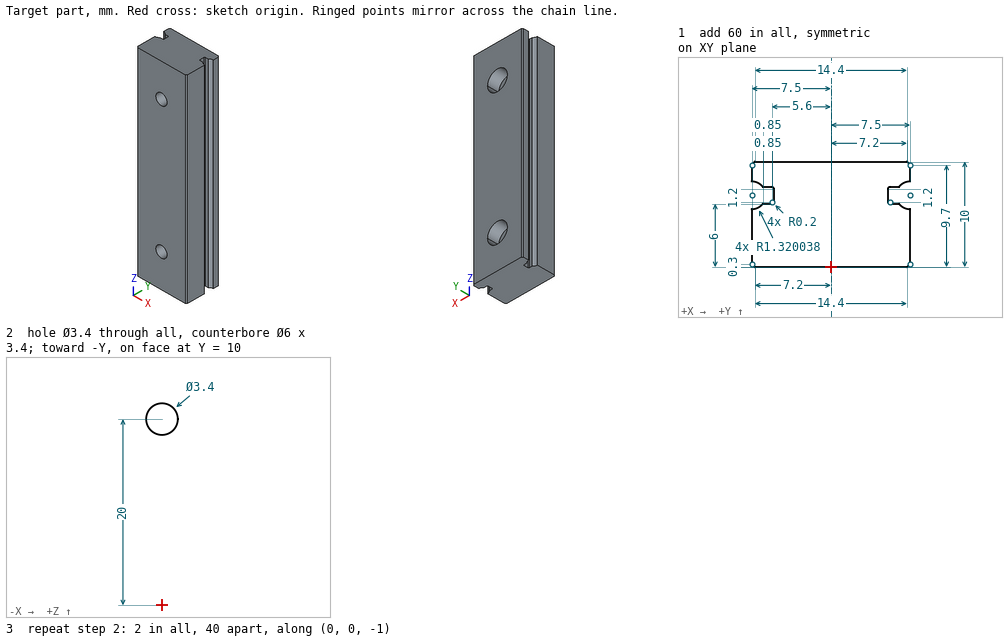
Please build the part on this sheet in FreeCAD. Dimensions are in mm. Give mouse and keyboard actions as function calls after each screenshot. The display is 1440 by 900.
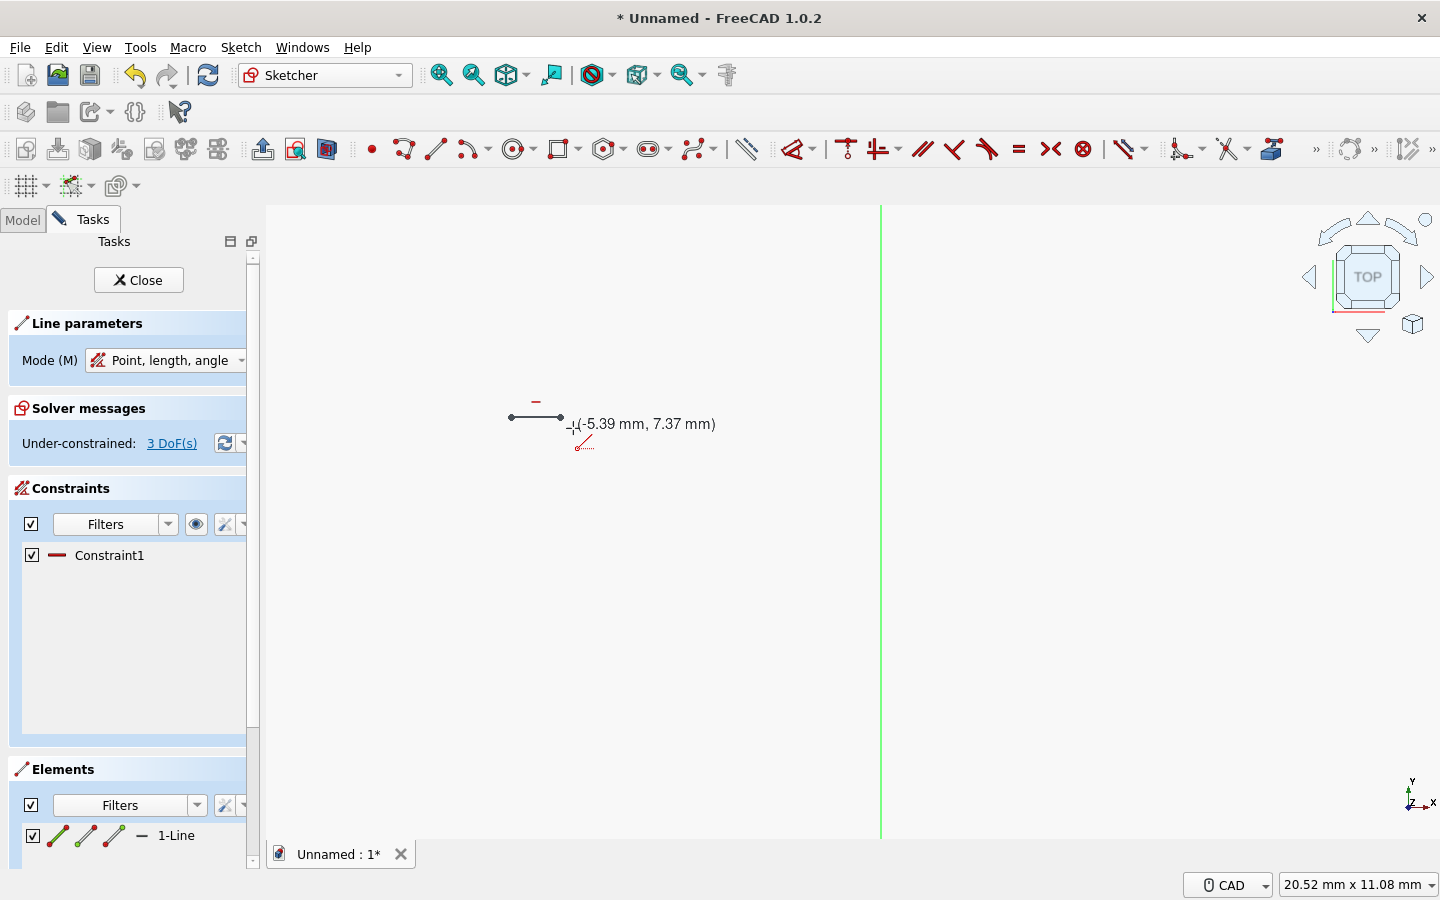
click(572, 428)
click(572, 496)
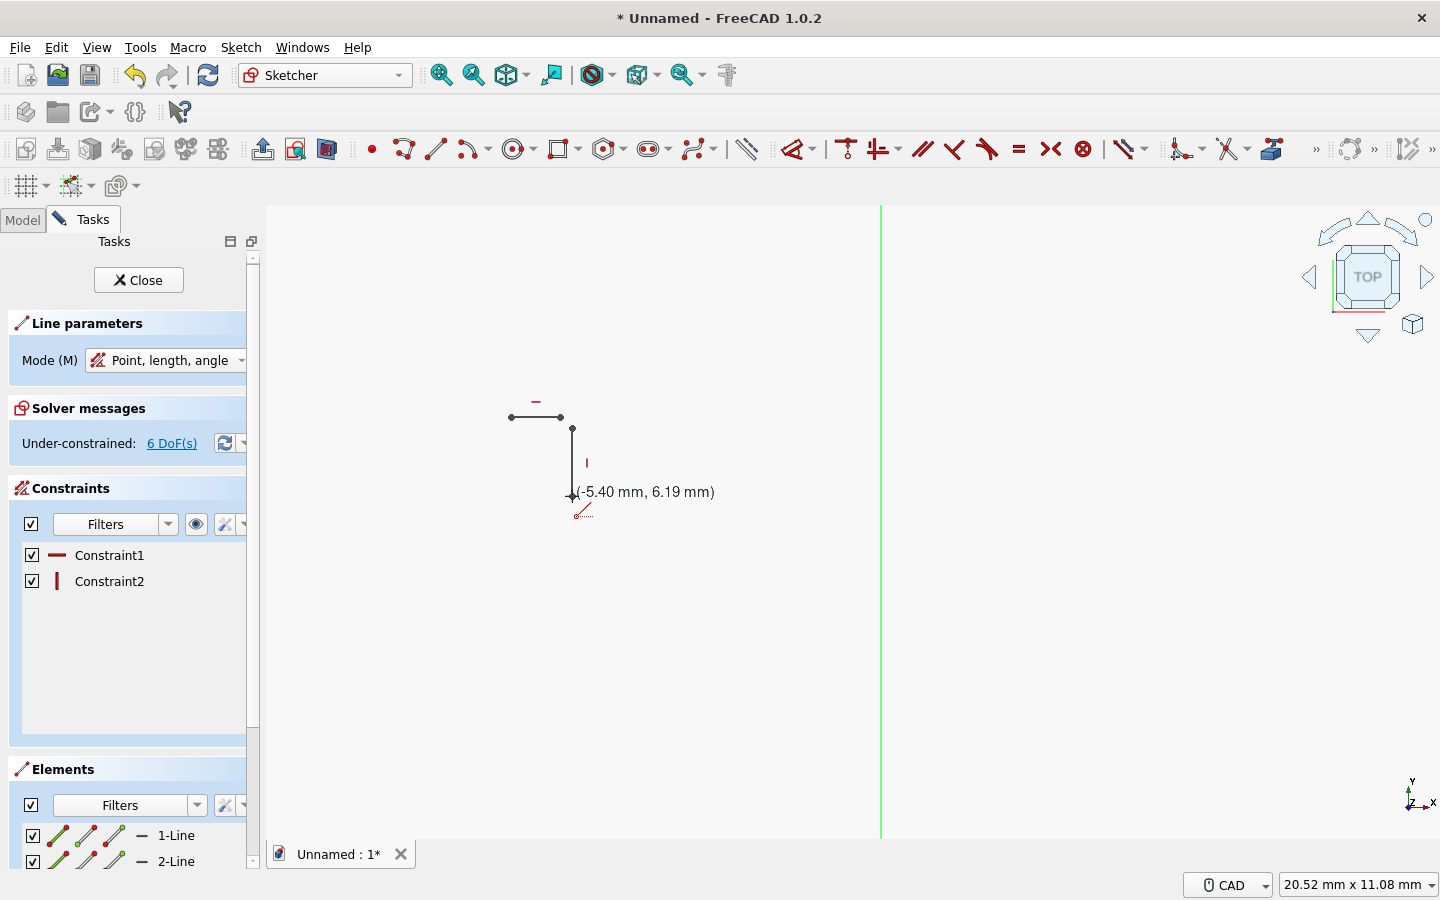
click(561, 508)
click(512, 508)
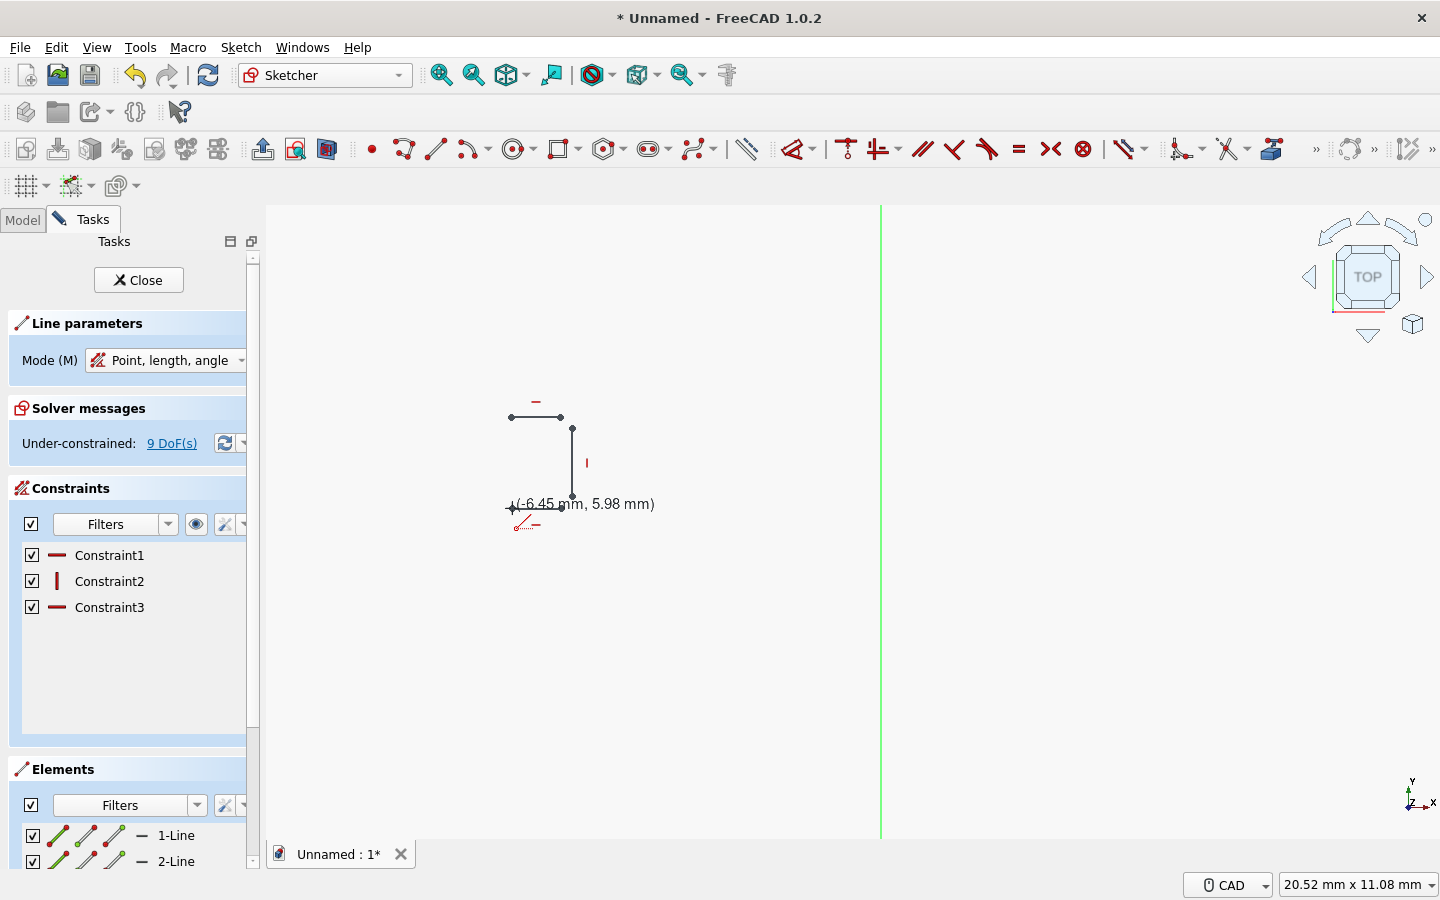
click(404, 150)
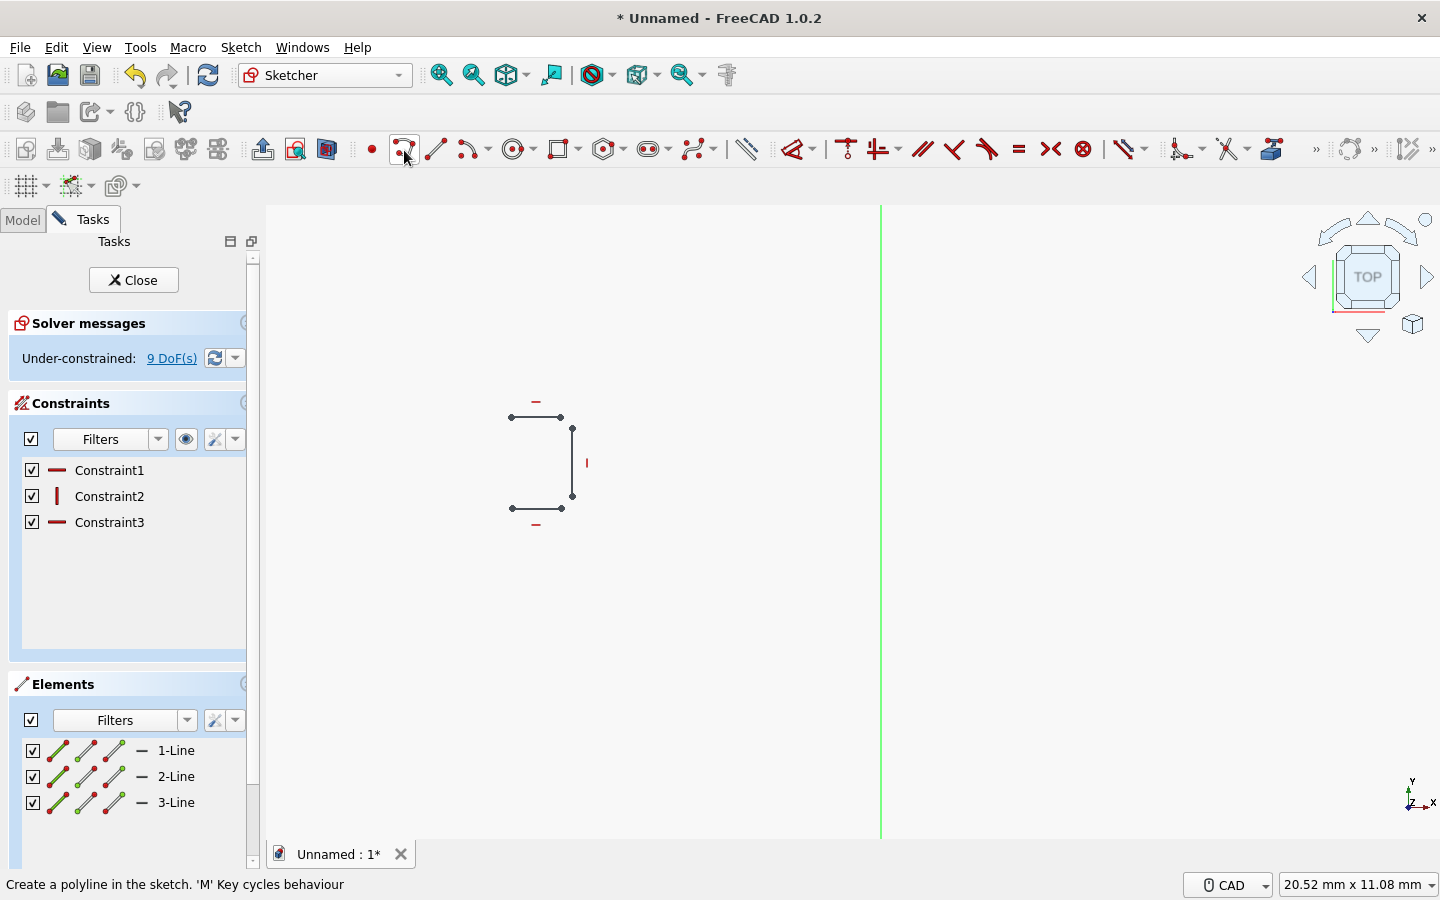
click(452, 537)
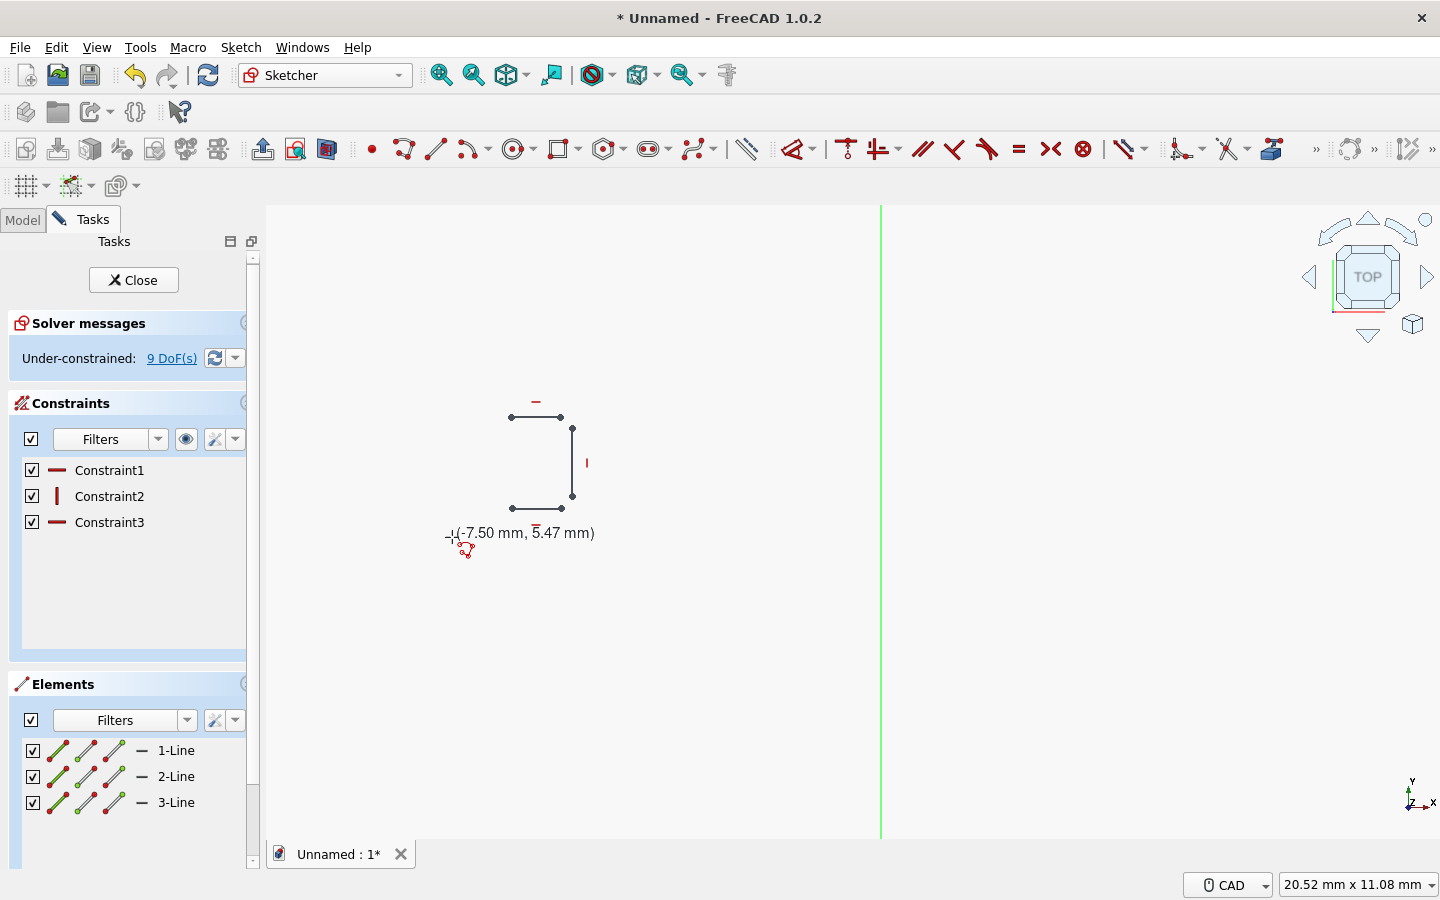
scroll(588, 435, down, 2)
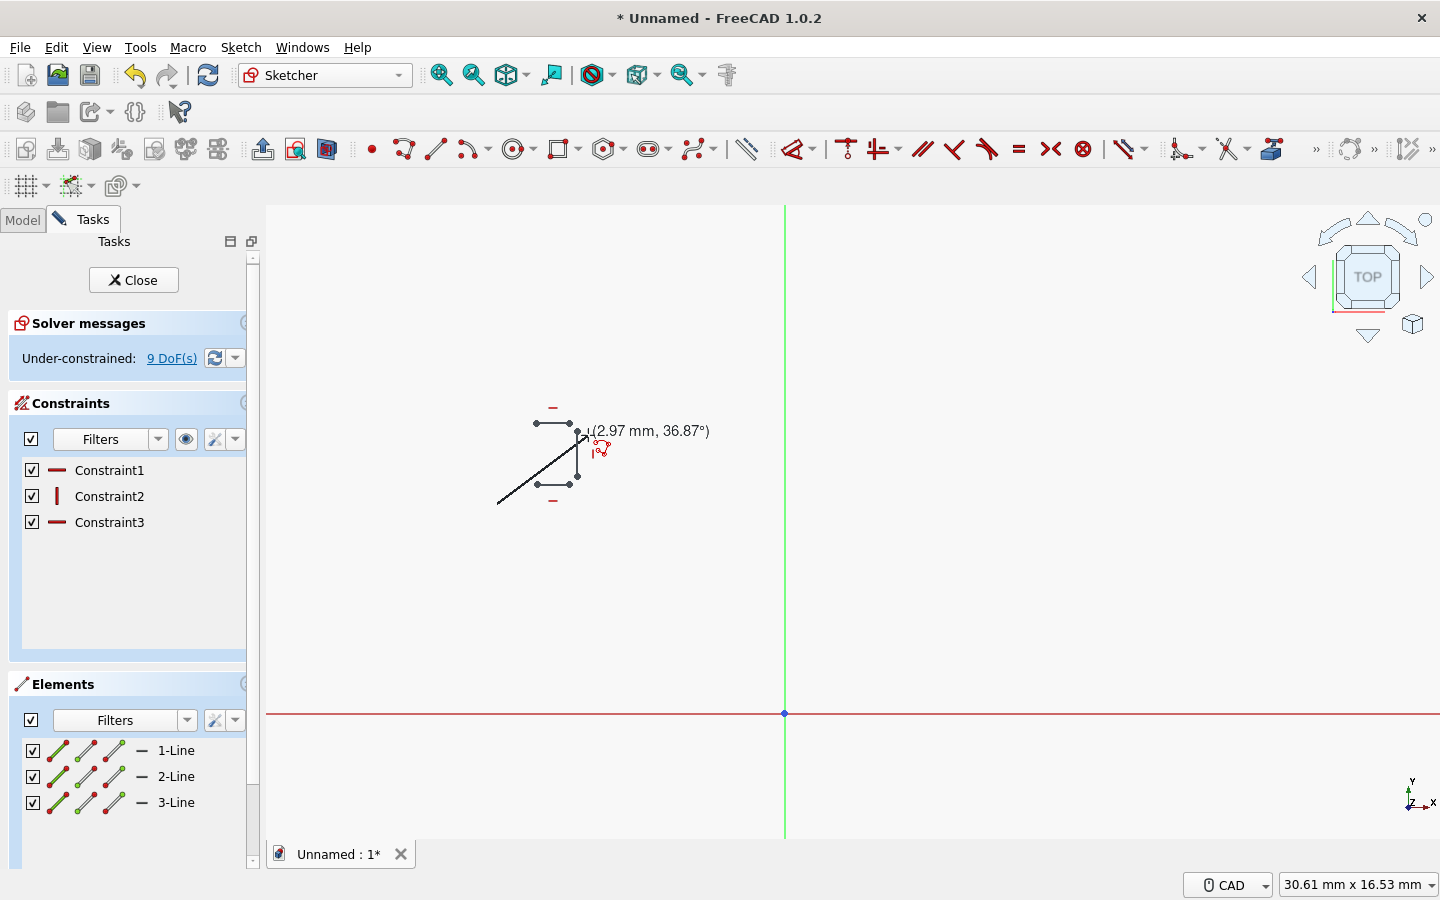
scroll(497, 702, up, 2)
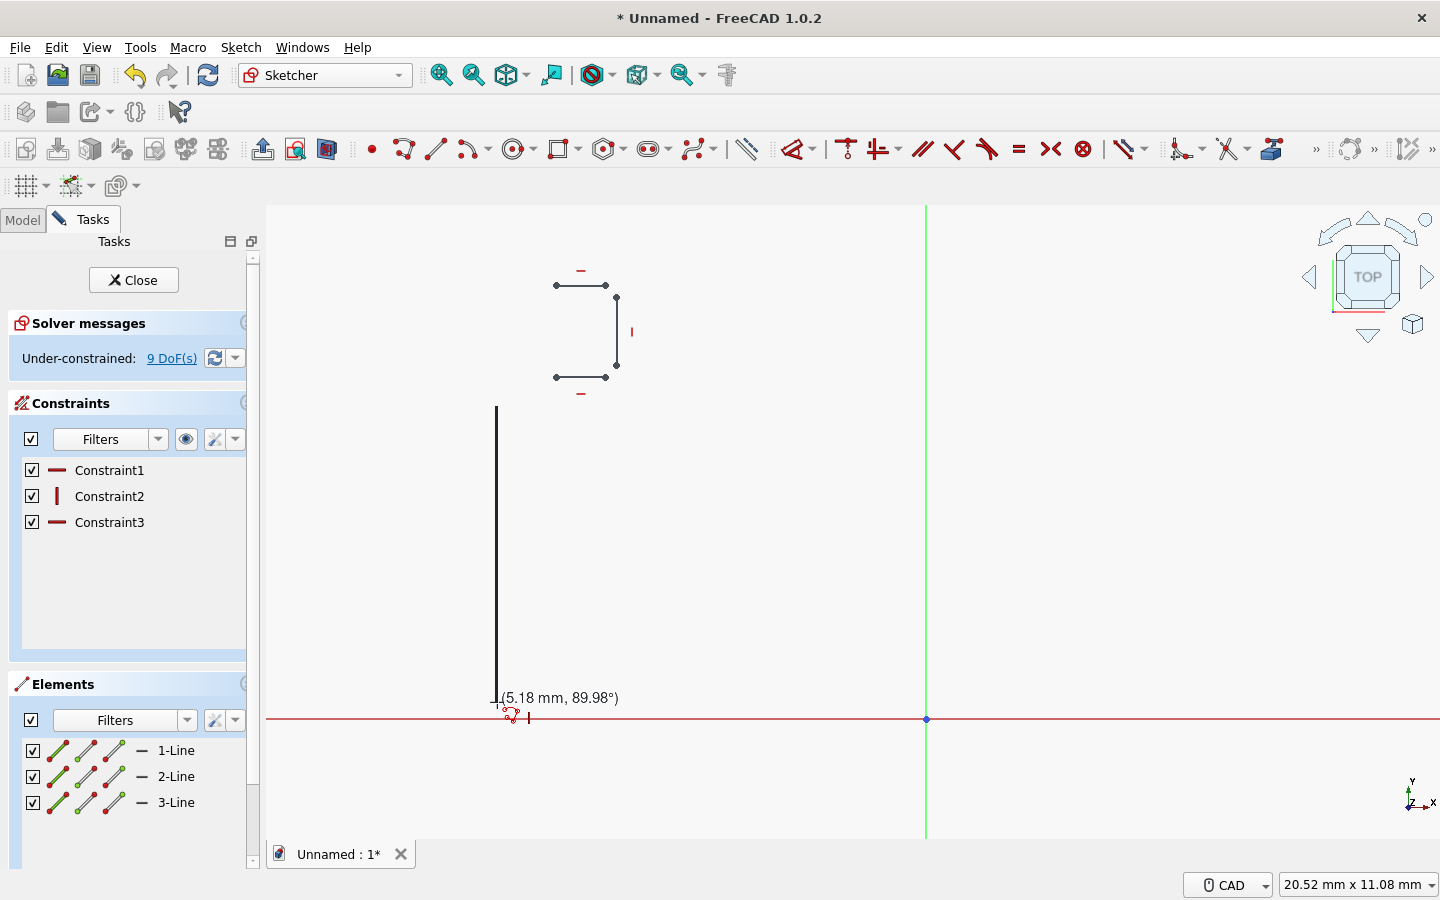
click(497, 702)
click(514, 719)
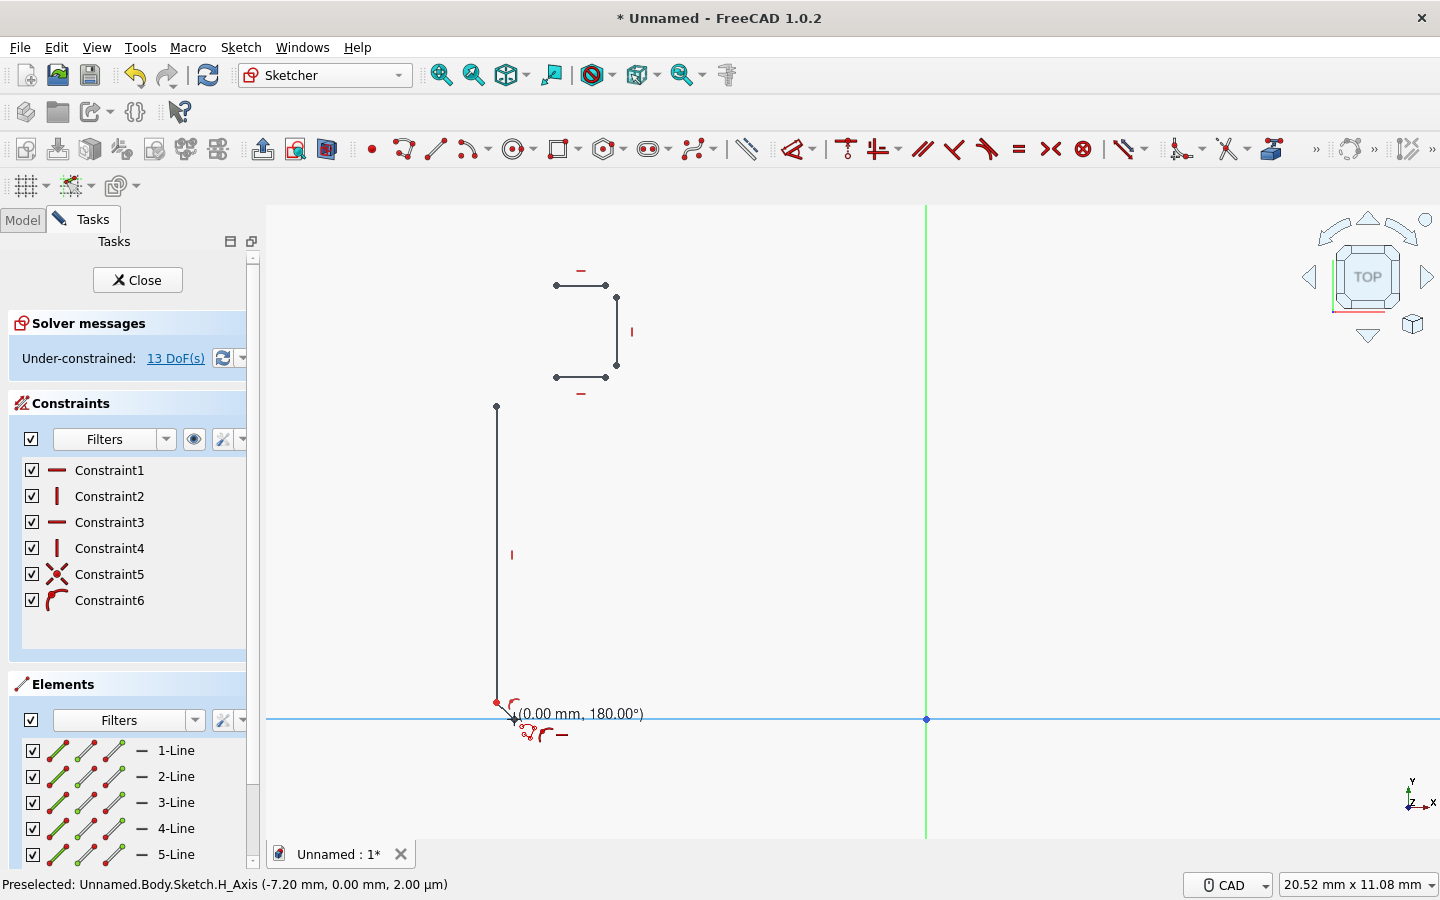
scroll(497, 702, down, 2)